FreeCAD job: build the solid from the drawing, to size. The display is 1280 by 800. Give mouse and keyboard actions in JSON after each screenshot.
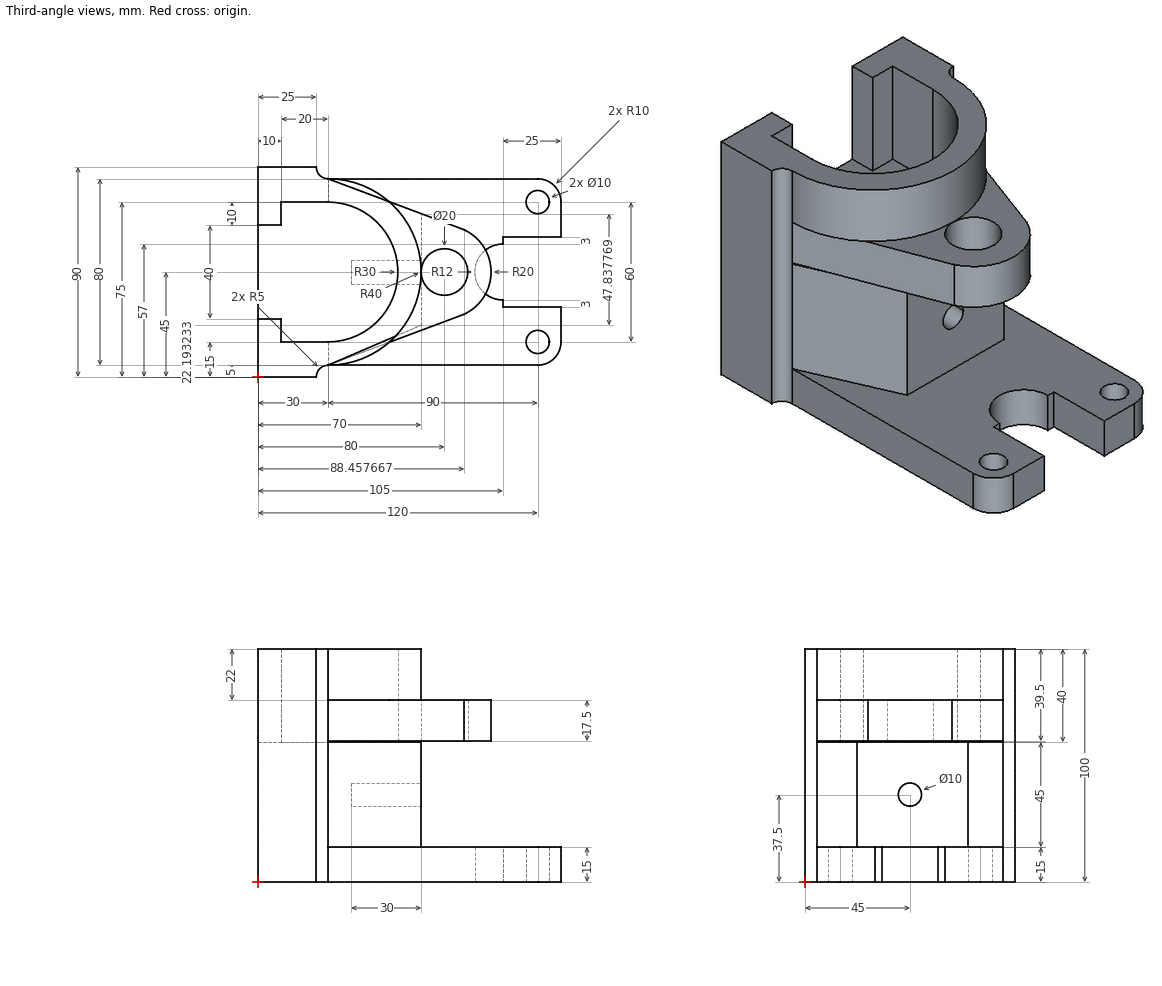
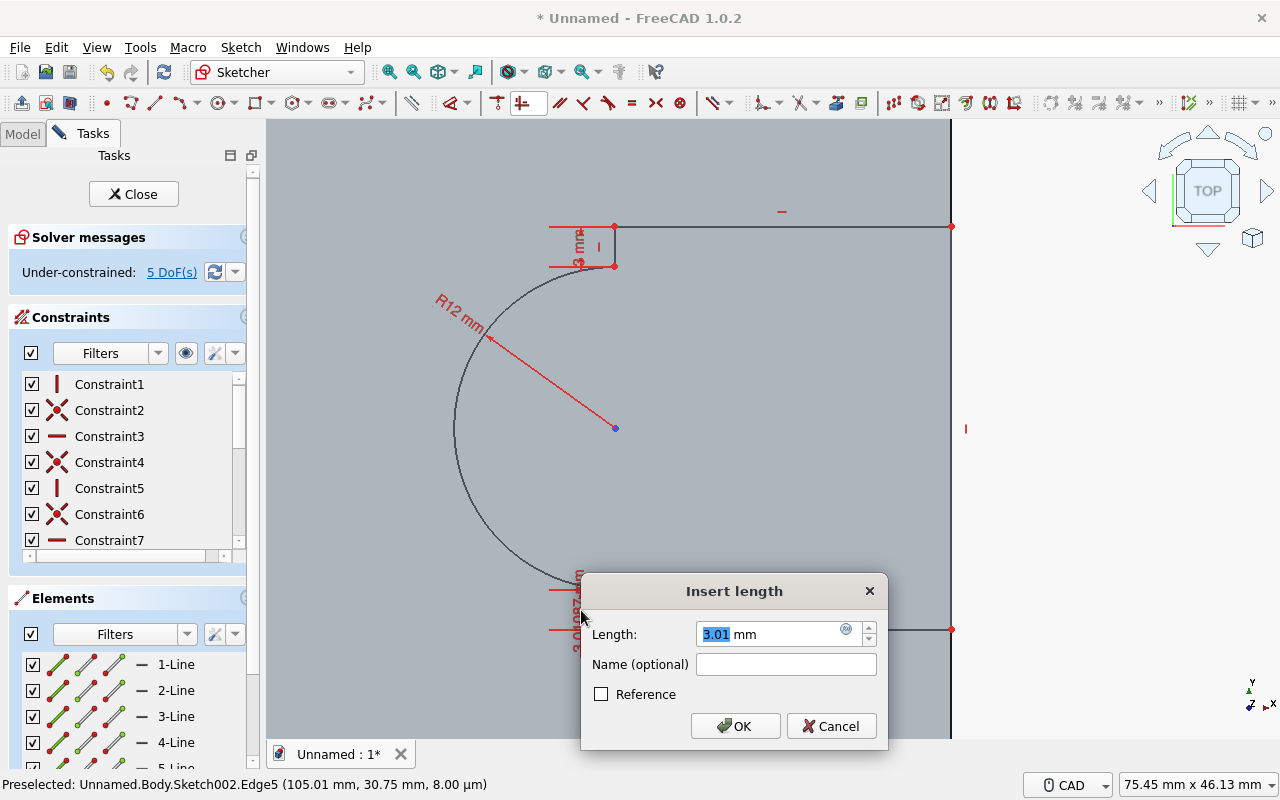
{"action": "type", "text": "3"}
{"action": "key", "text": "Return"}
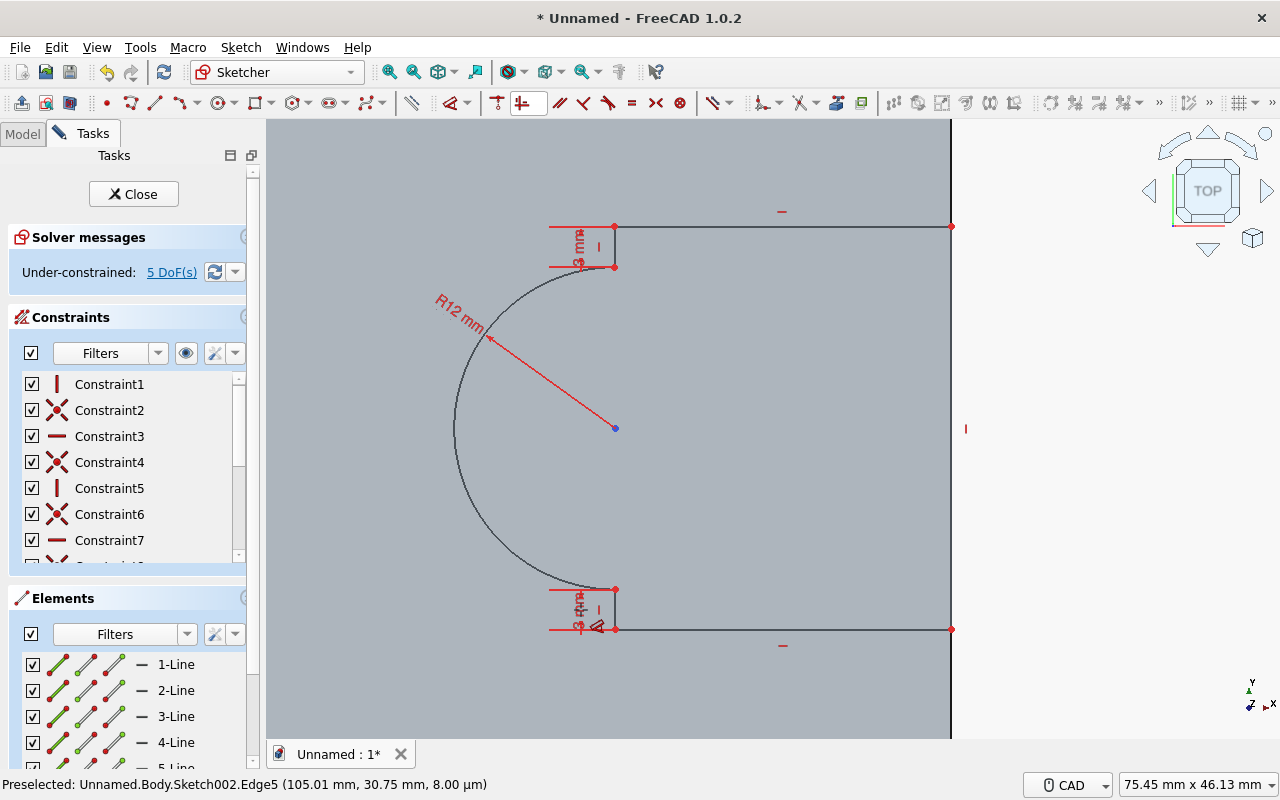
{"action": "left_click", "coordinate": [716, 227]}
{"action": "left_click", "coordinate": [783, 193]}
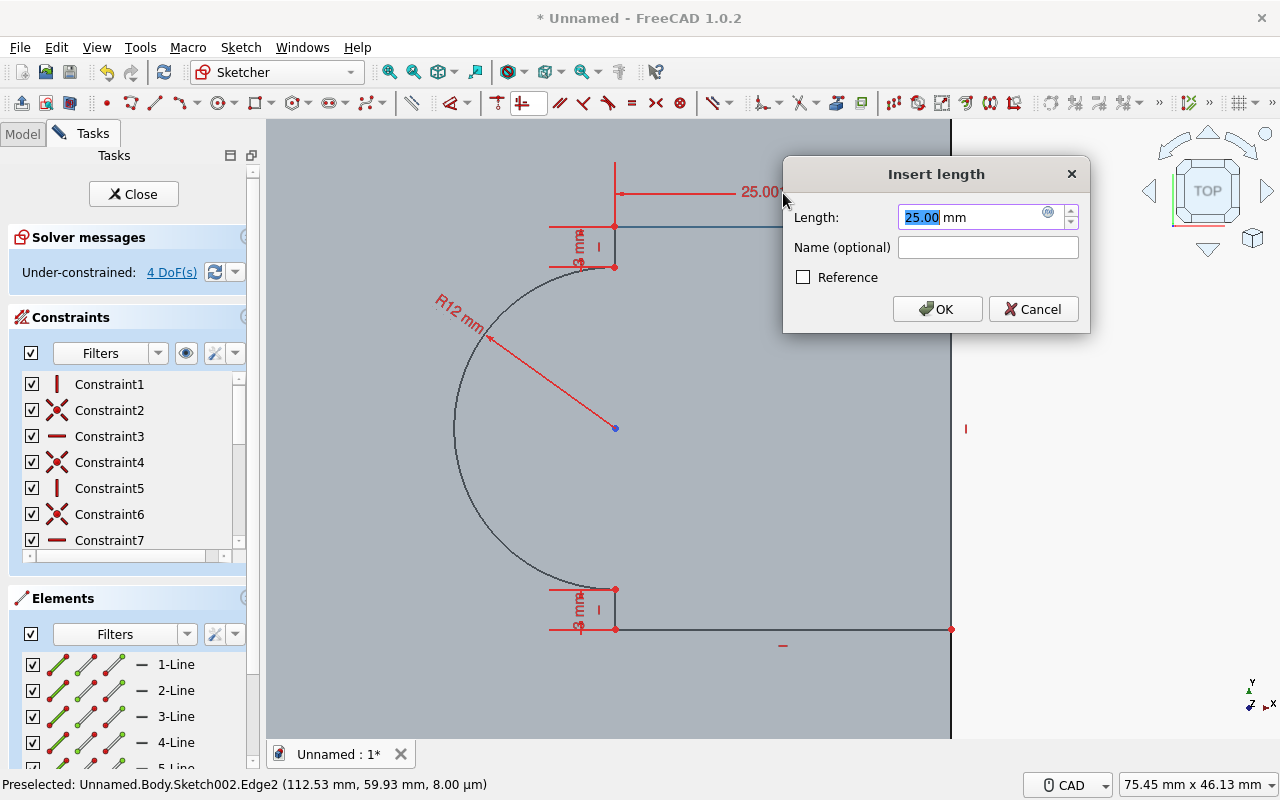
{"action": "type", "text": "25"}
{"action": "key", "text": "Return"}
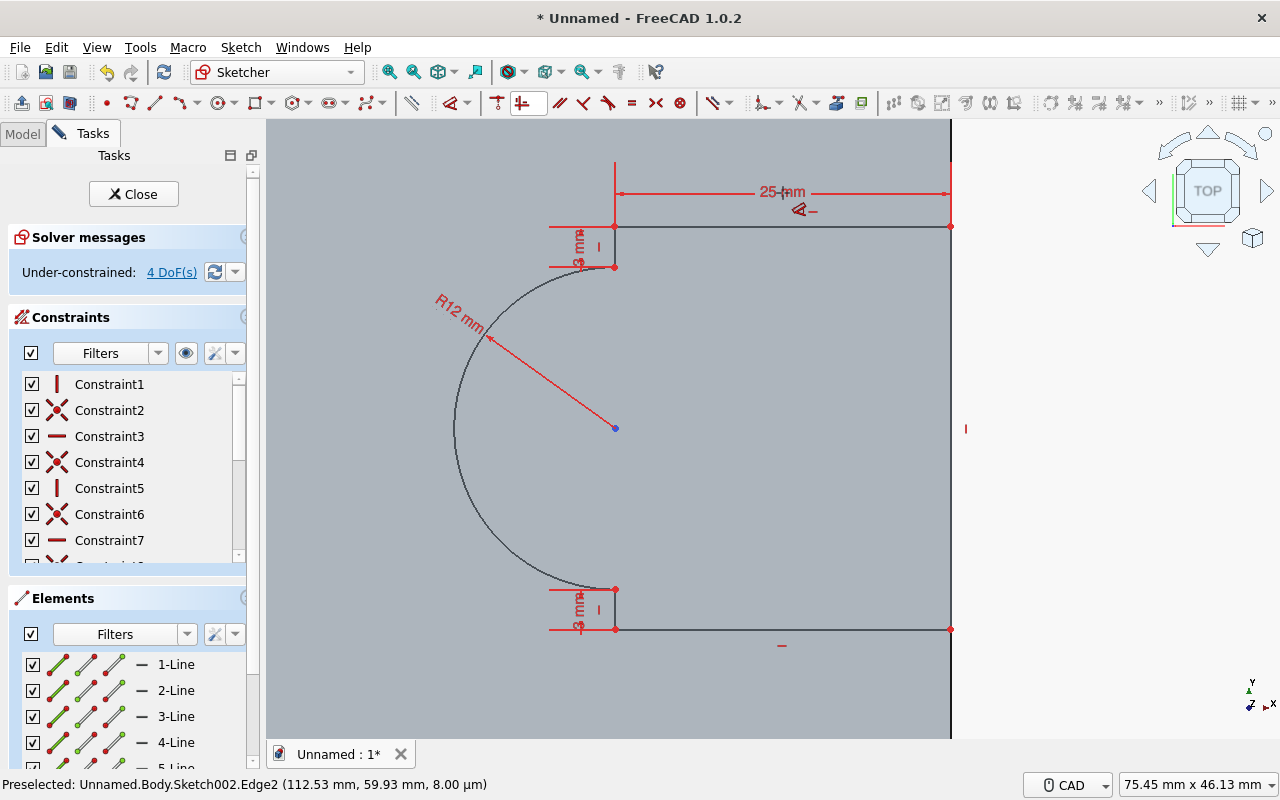
{"action": "left_click", "coordinate": [850, 630]}
{"action": "left_click", "coordinate": [783, 664]}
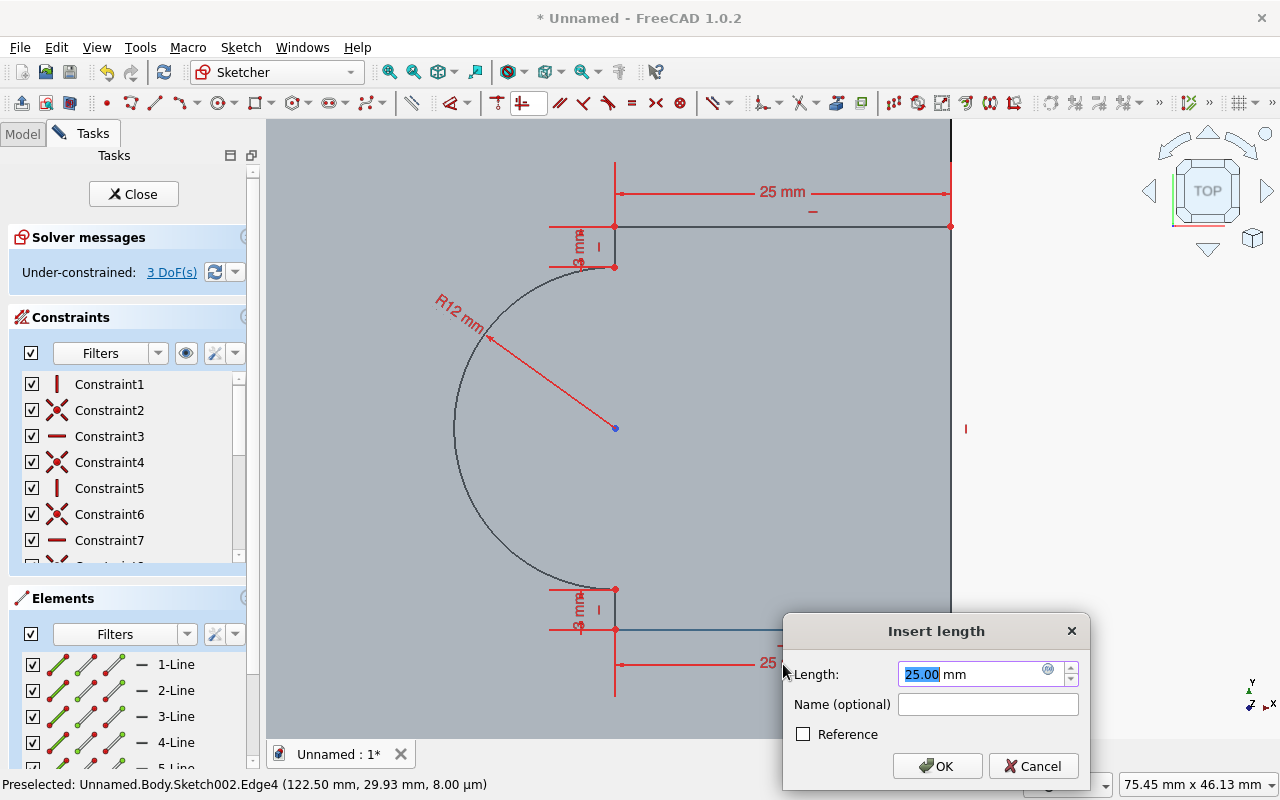
{"action": "type", "text": "25"}
{"action": "key", "text": "Return"}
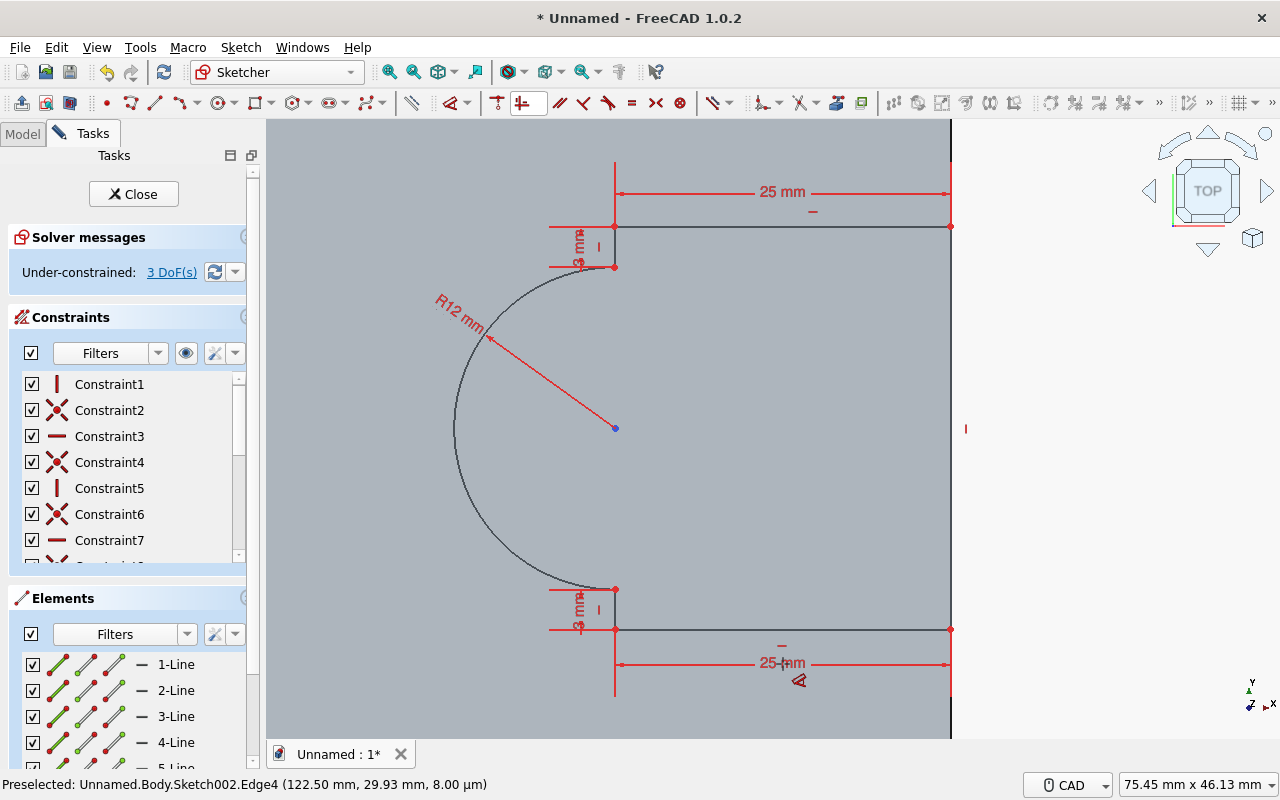
{"action": "left_click", "coordinate": [615, 267]}
{"action": "left_click", "coordinate": [649, 489]}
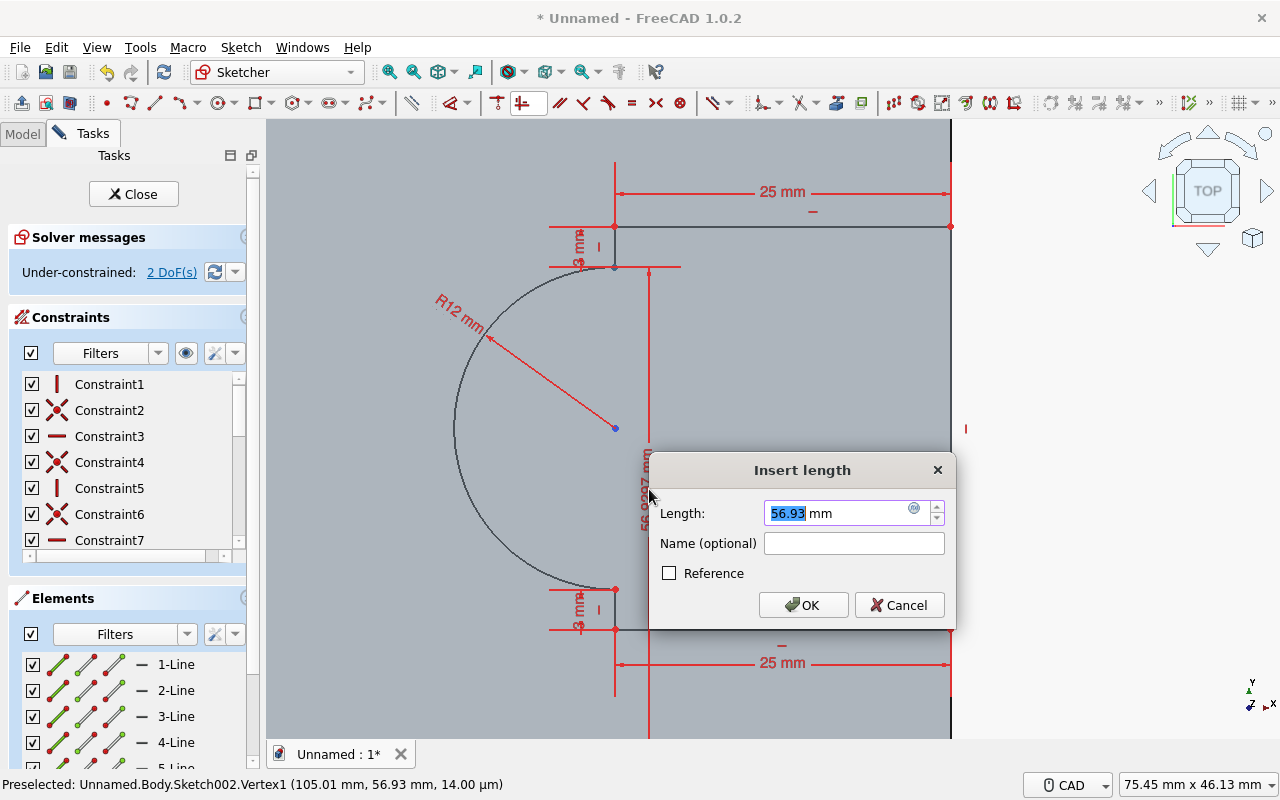
{"action": "type", "text": "57"}
{"action": "key", "text": "Return"}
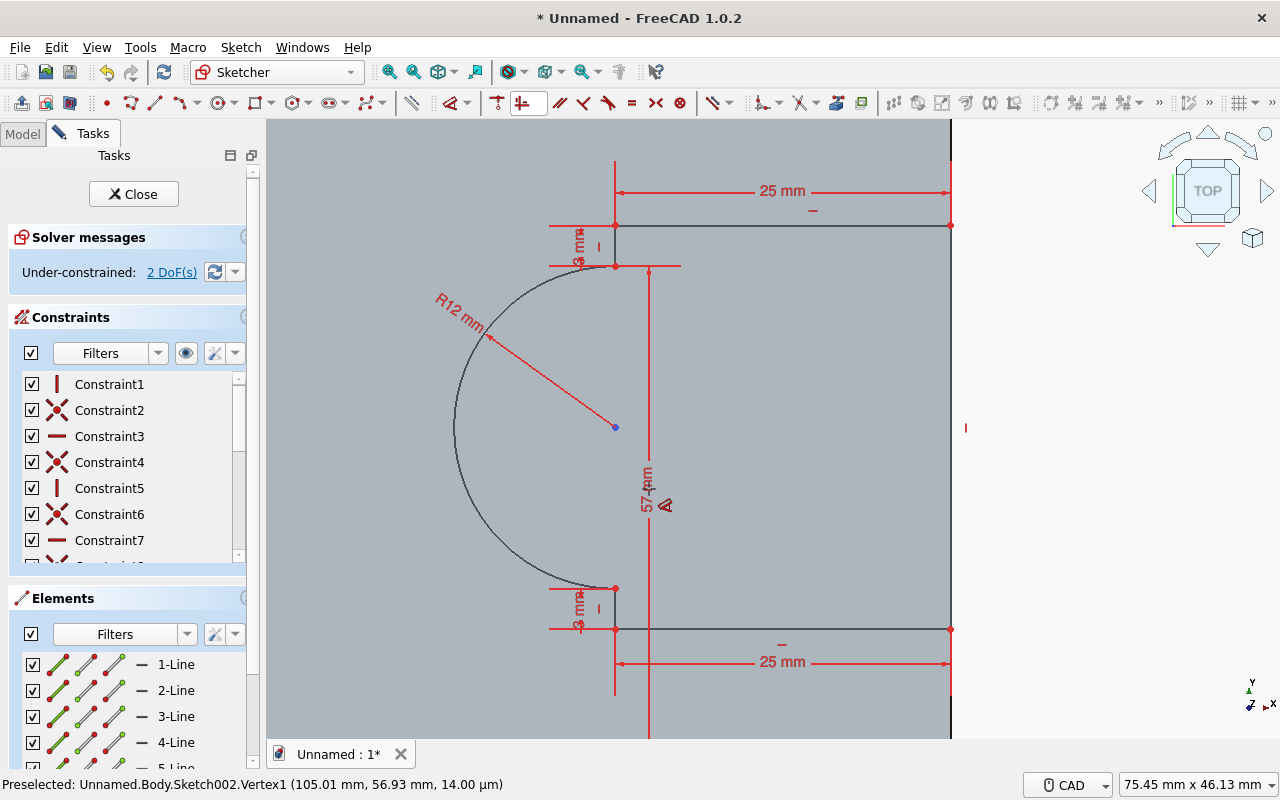
{"action": "left_click", "coordinate": [615, 266]}
{"action": "left_click", "coordinate": [454, 232]}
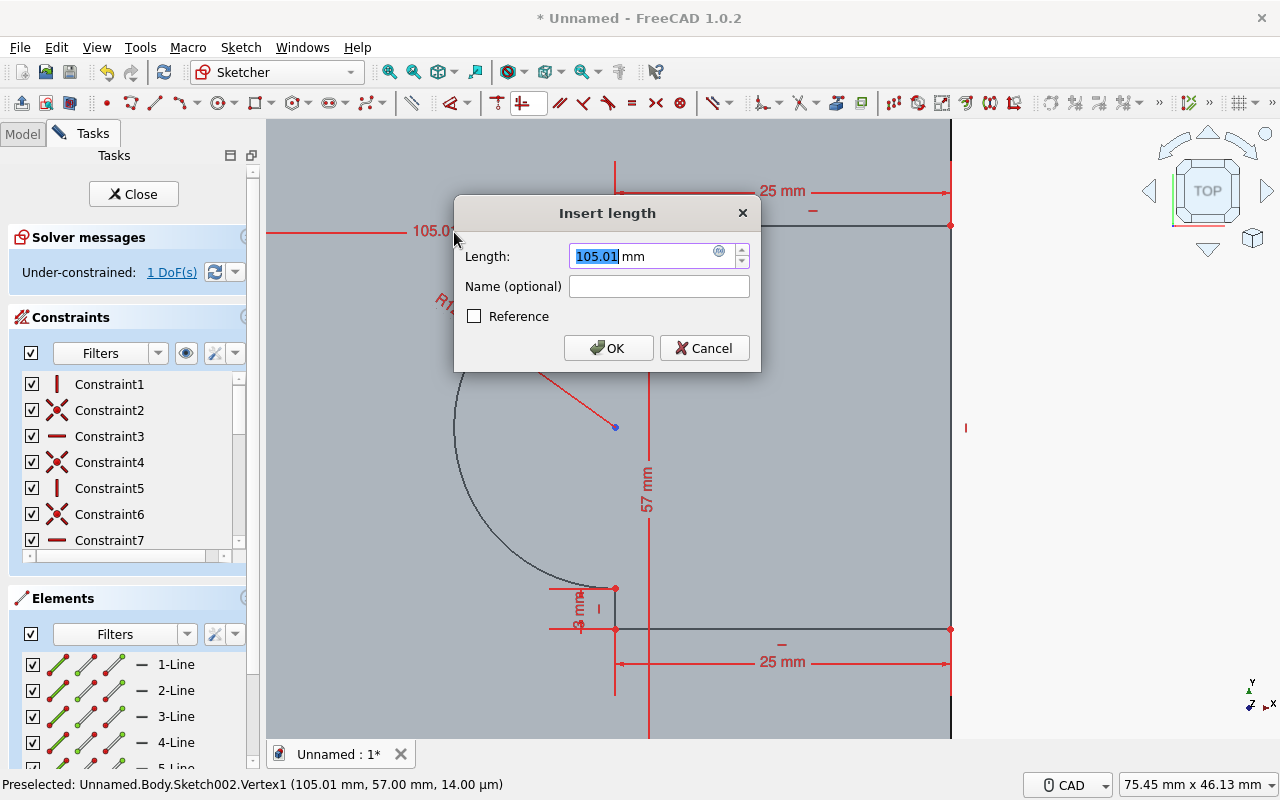
{"action": "type", "text": "105"}
{"action": "key", "text": "Return"}